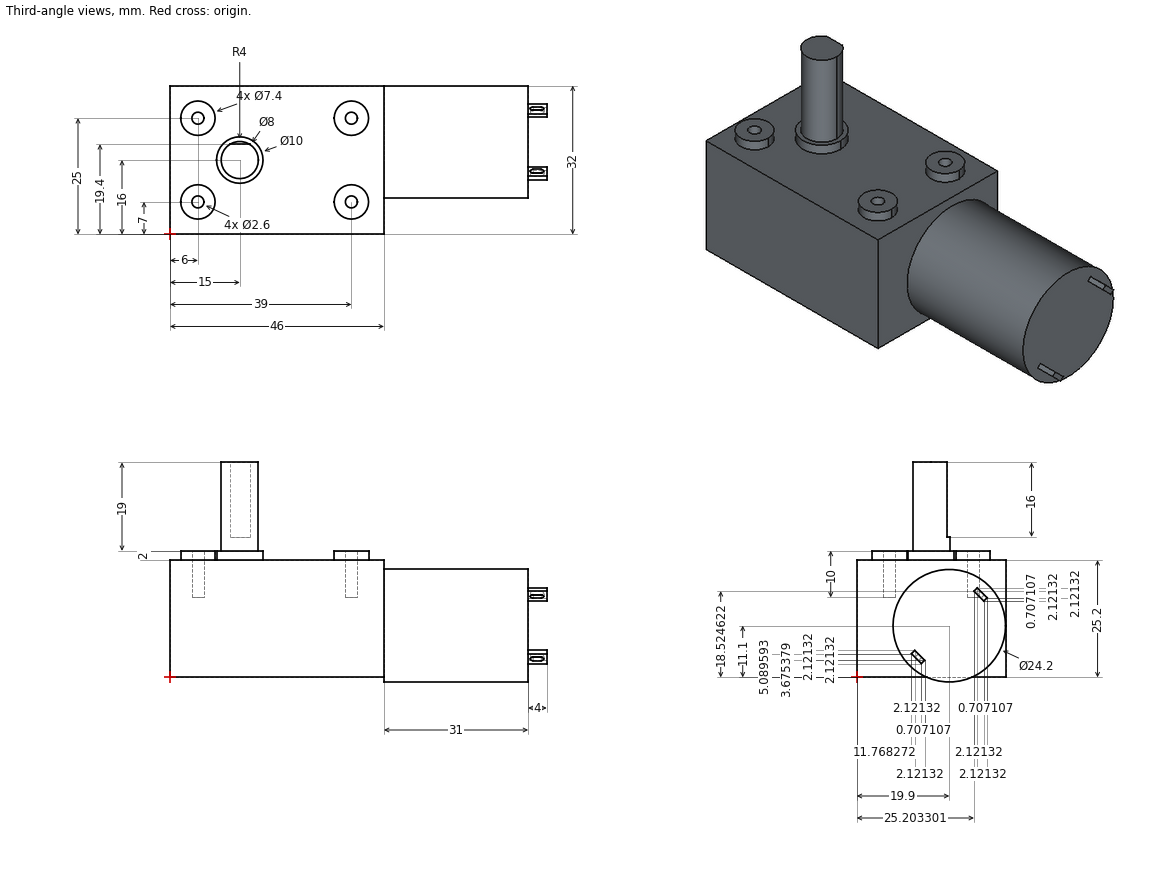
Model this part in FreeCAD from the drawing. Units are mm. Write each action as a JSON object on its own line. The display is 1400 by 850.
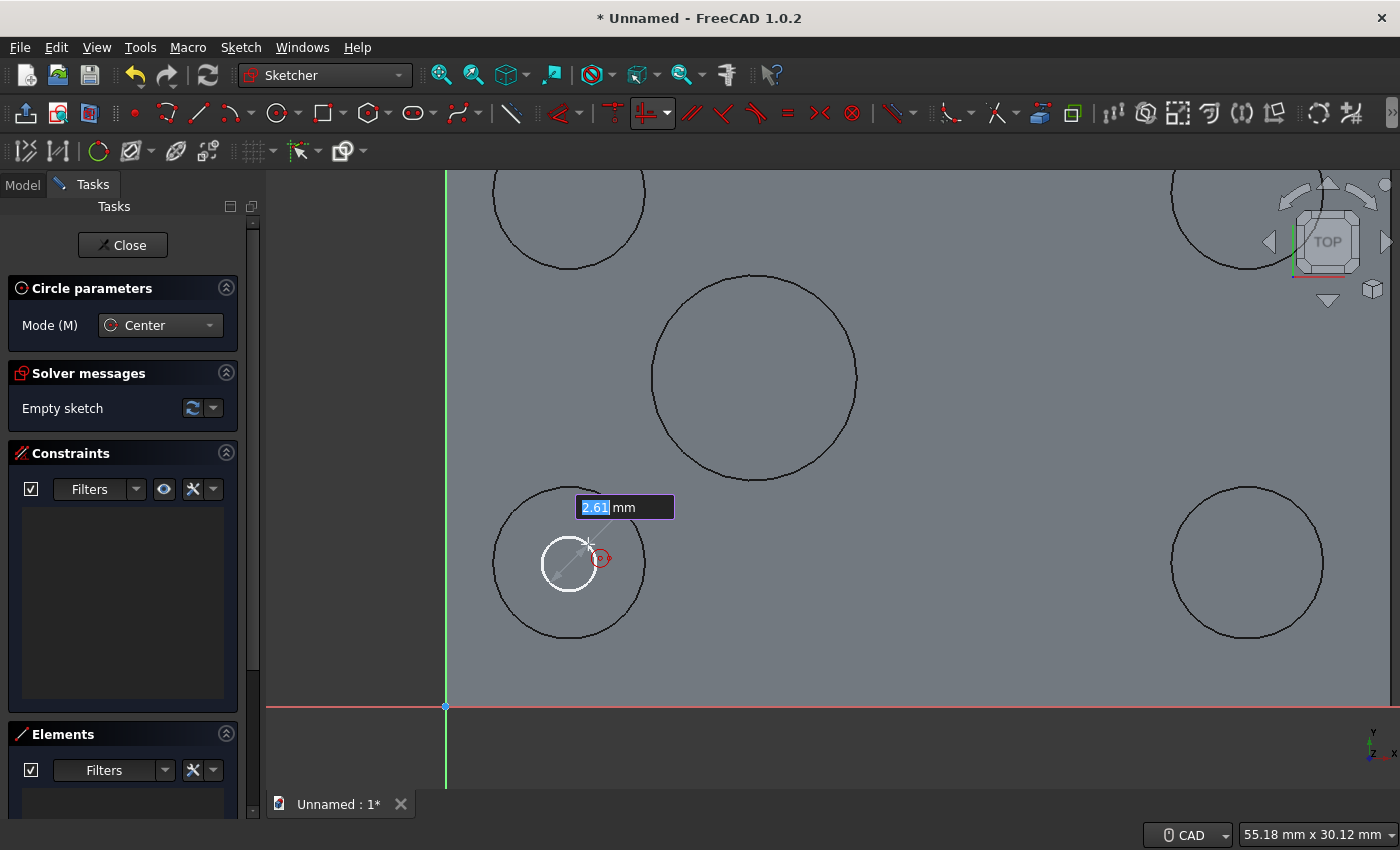
{"action": "type", "text": "2.6"}
{"action": "key", "text": "Return"}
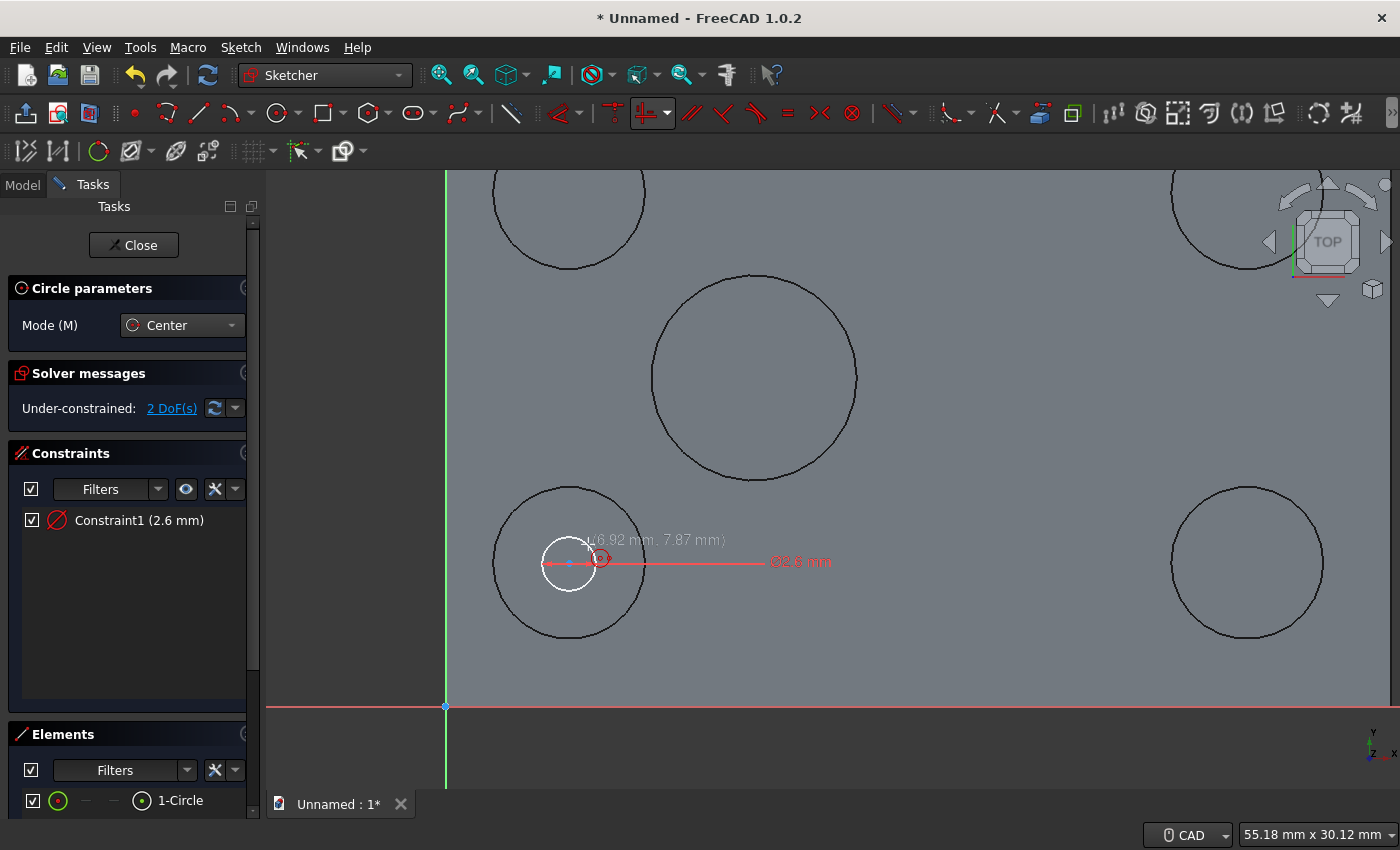
{"action": "scroll", "coordinate": [571, 567], "scroll_direction": "down", "scroll_amount": 2}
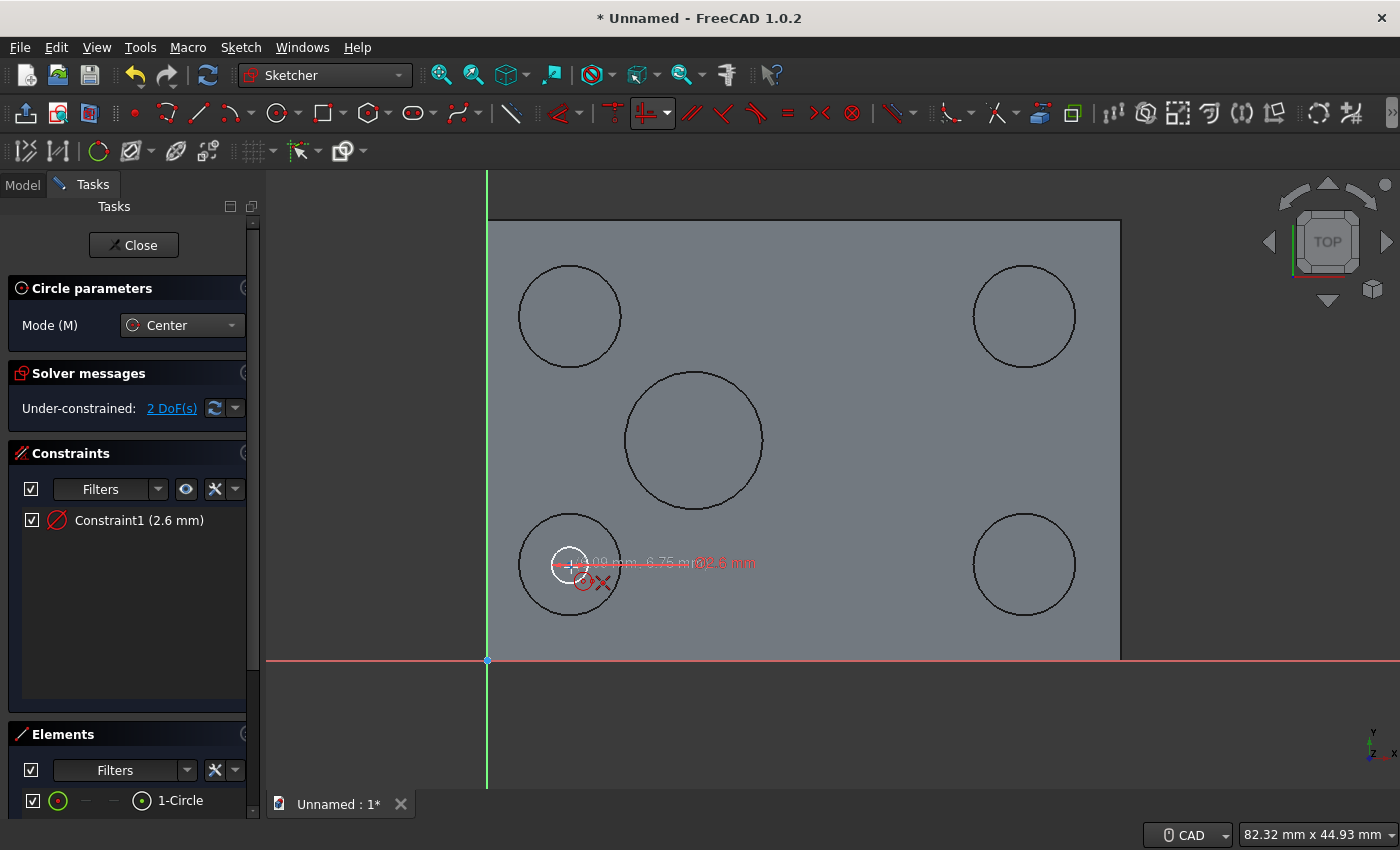
{"action": "scroll", "coordinate": [570, 317], "scroll_direction": "up", "scroll_amount": 2}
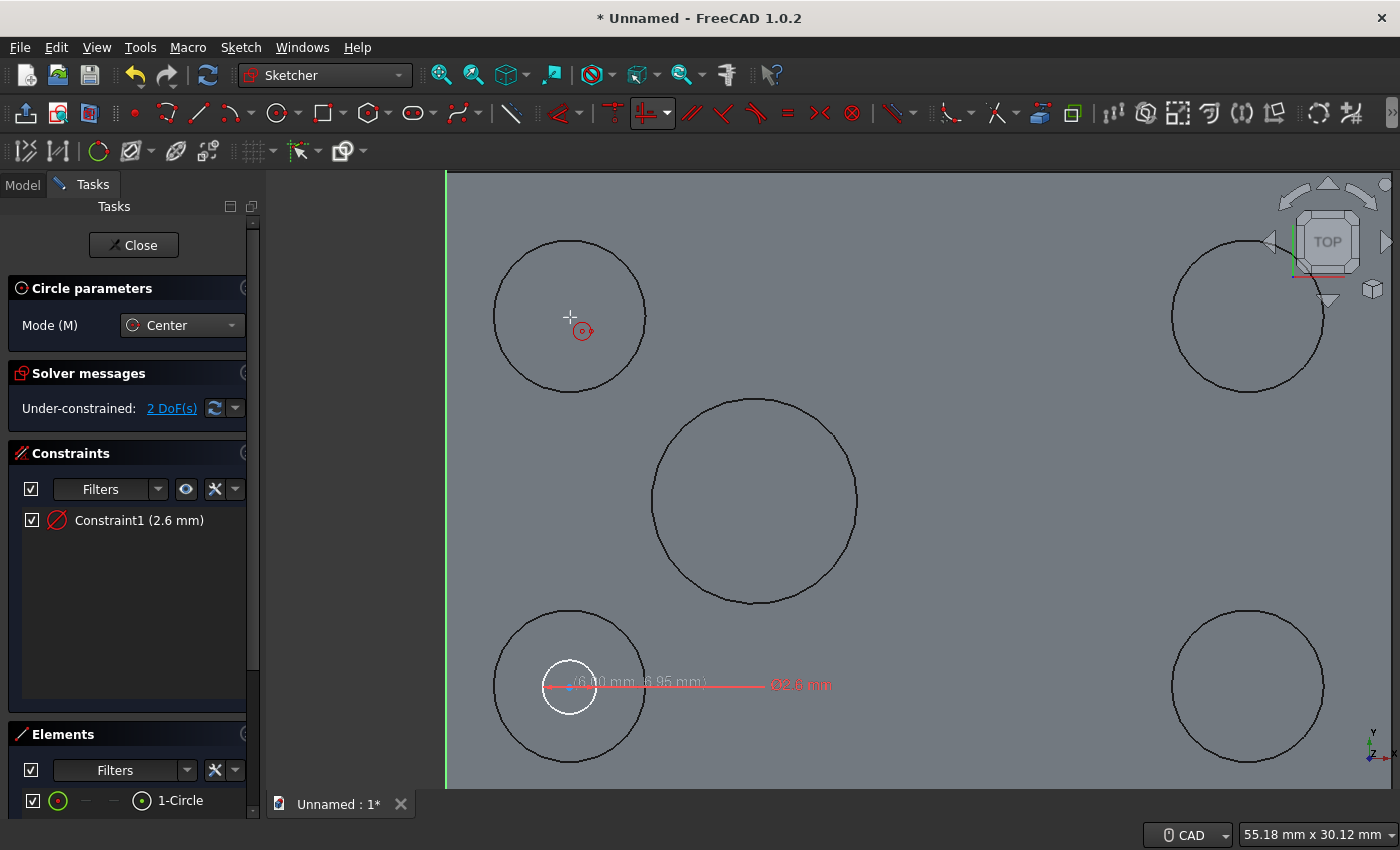
{"action": "left_click", "coordinate": [570, 316]}
{"action": "mouse_move", "coordinate": [588, 297]}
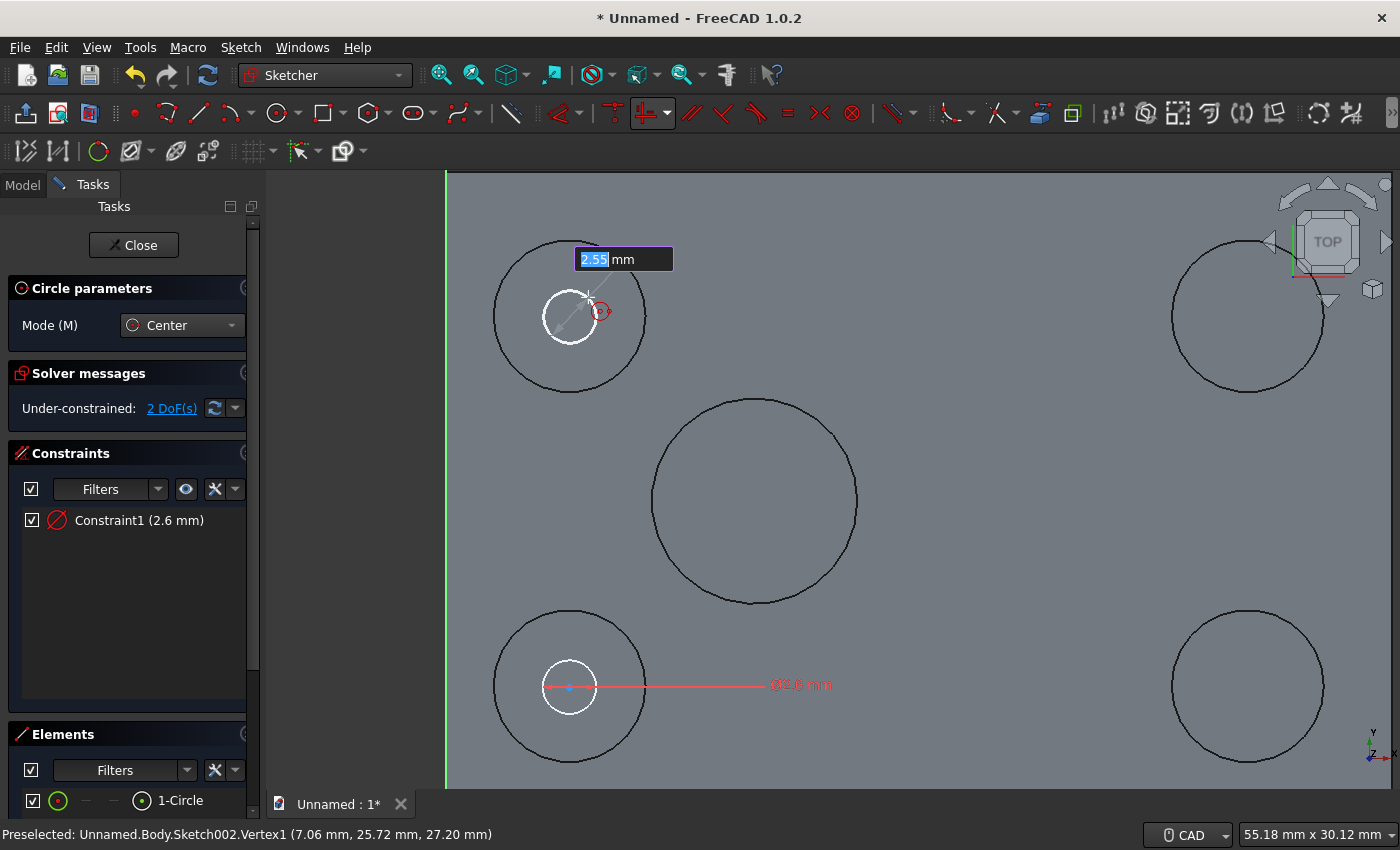
{"action": "type", "text": "2.6"}
{"action": "key", "text": "Return"}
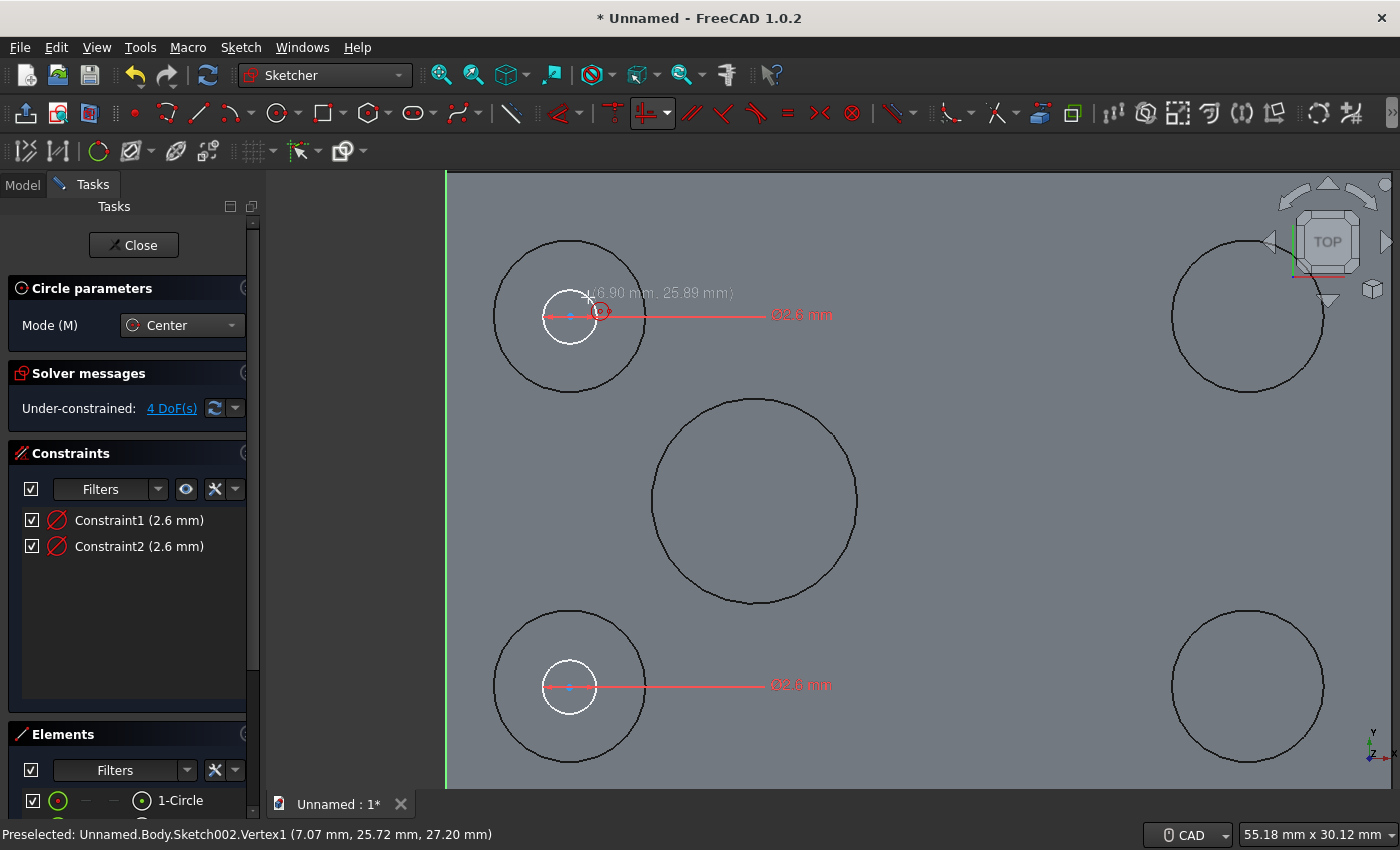
{"action": "scroll", "coordinate": [570, 316], "scroll_direction": "down", "scroll_amount": 2}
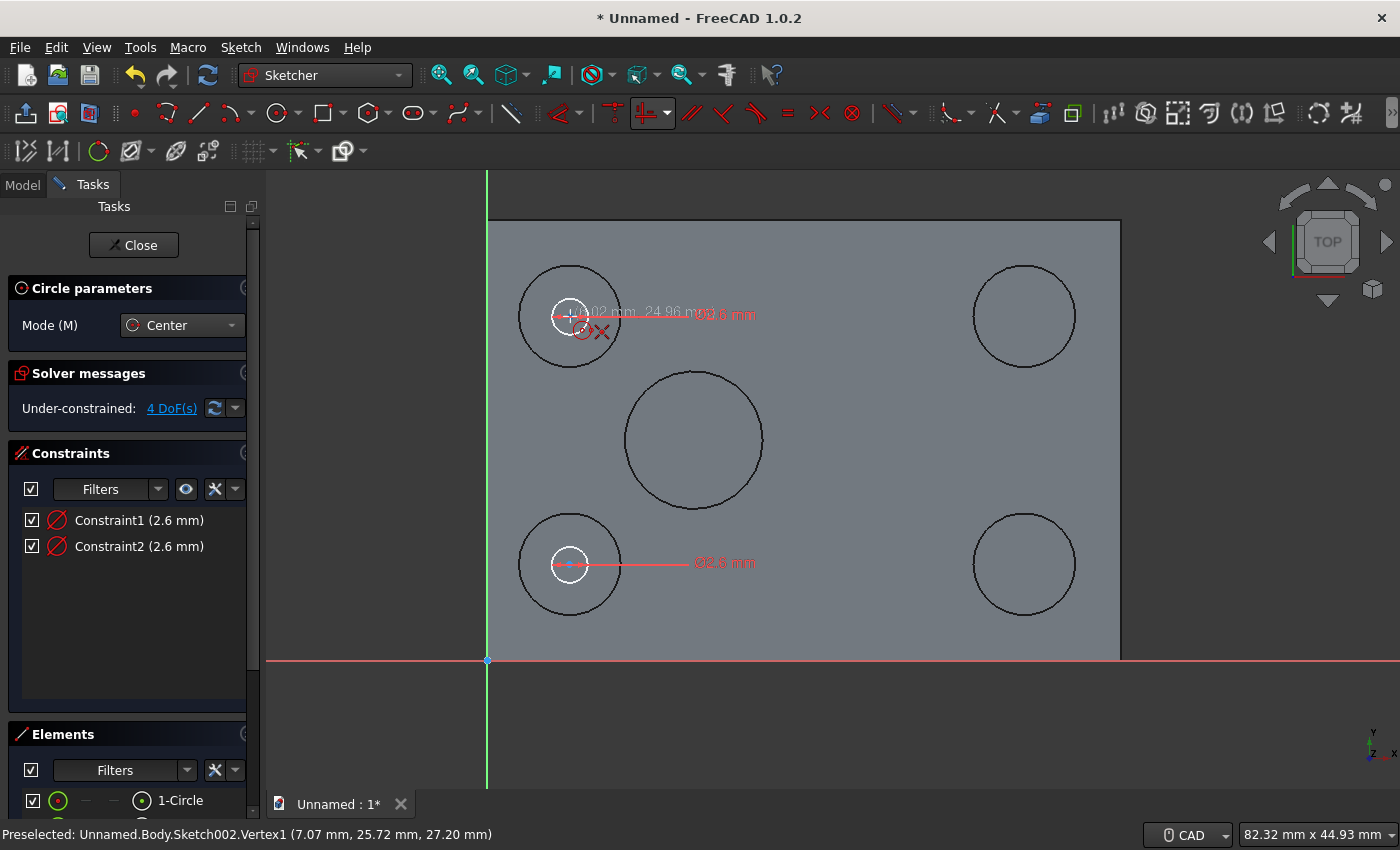
{"action": "scroll", "coordinate": [1024, 316], "scroll_direction": "up", "scroll_amount": 2}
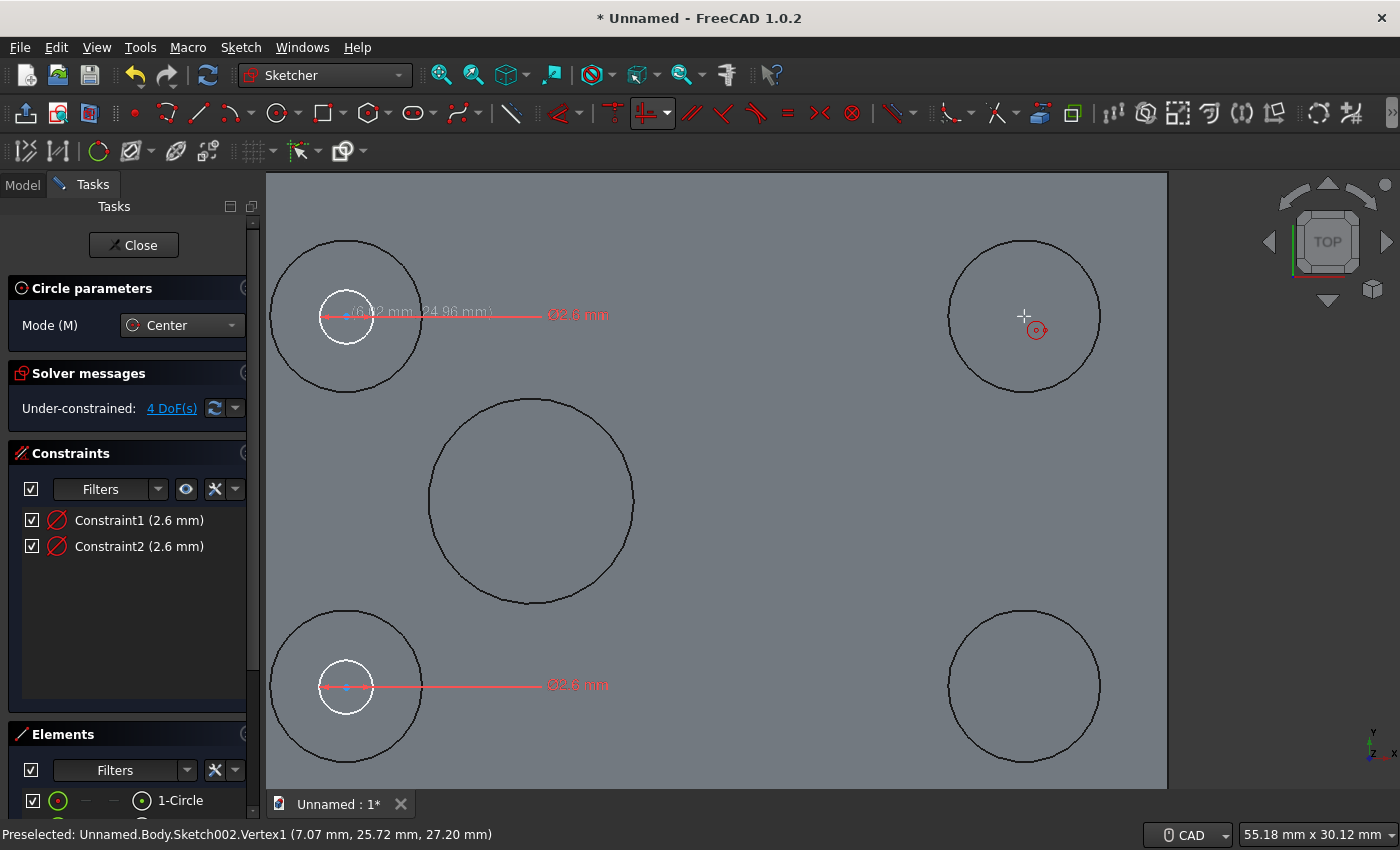
{"action": "left_click", "coordinate": [1024, 316]}
{"action": "mouse_move", "coordinate": [1043, 297]}